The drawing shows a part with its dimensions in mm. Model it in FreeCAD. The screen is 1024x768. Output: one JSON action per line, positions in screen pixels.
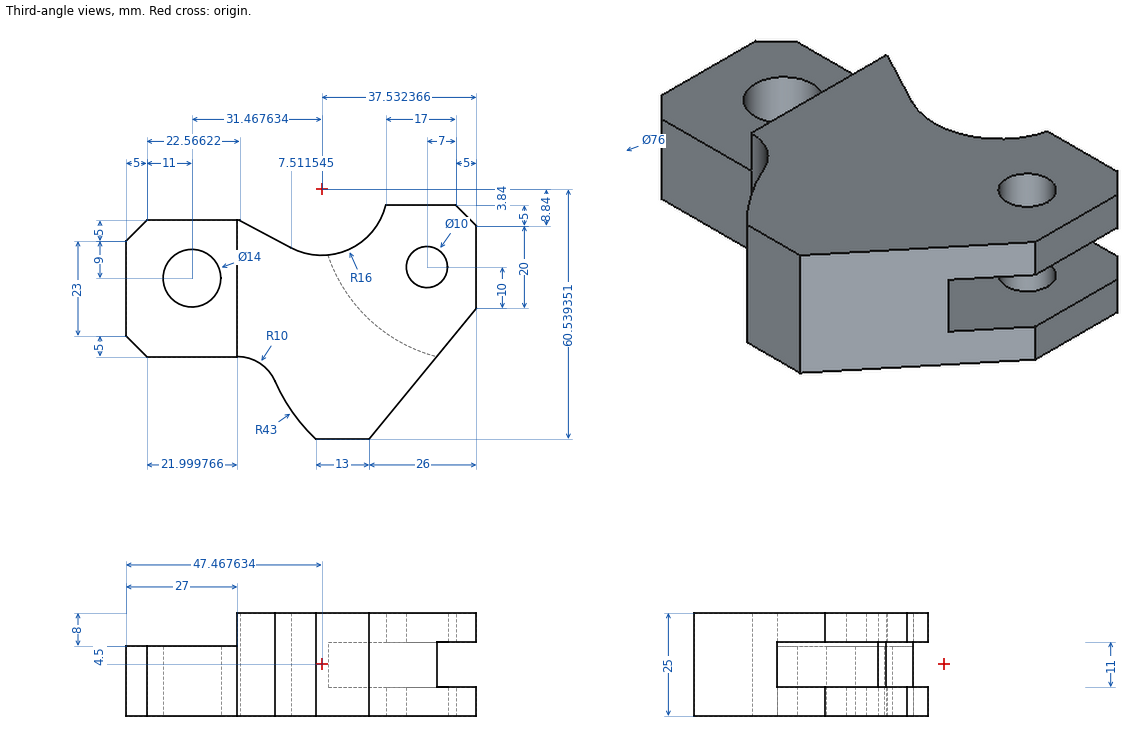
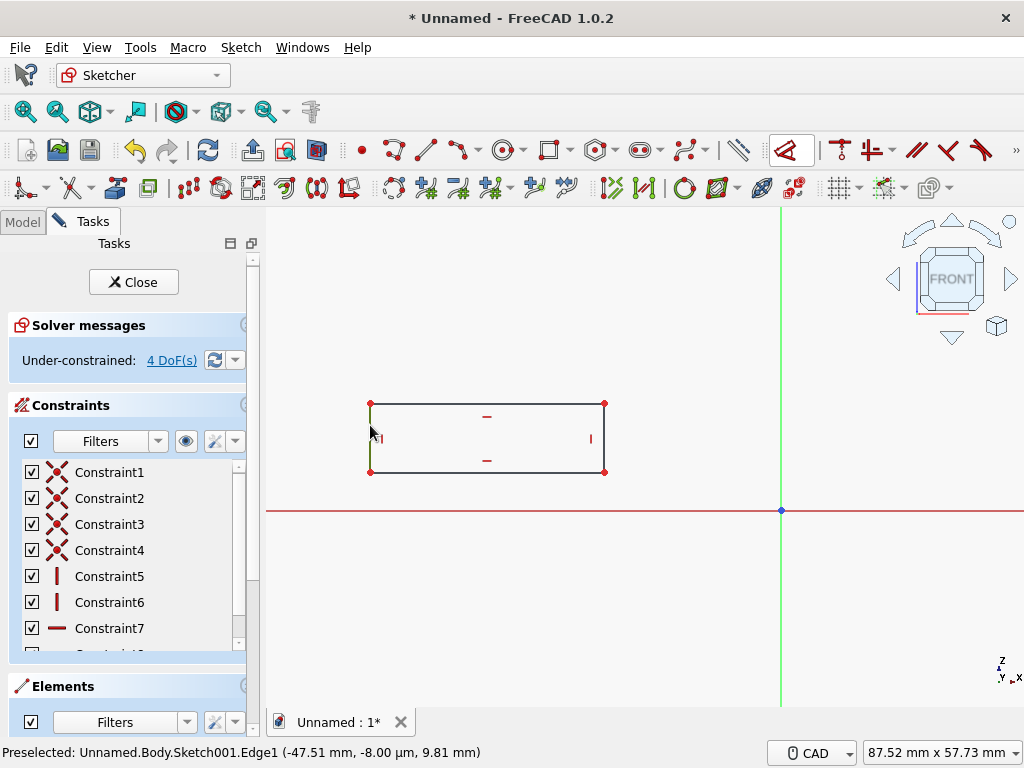
{"action": "left_click", "coordinate": [808, 150]}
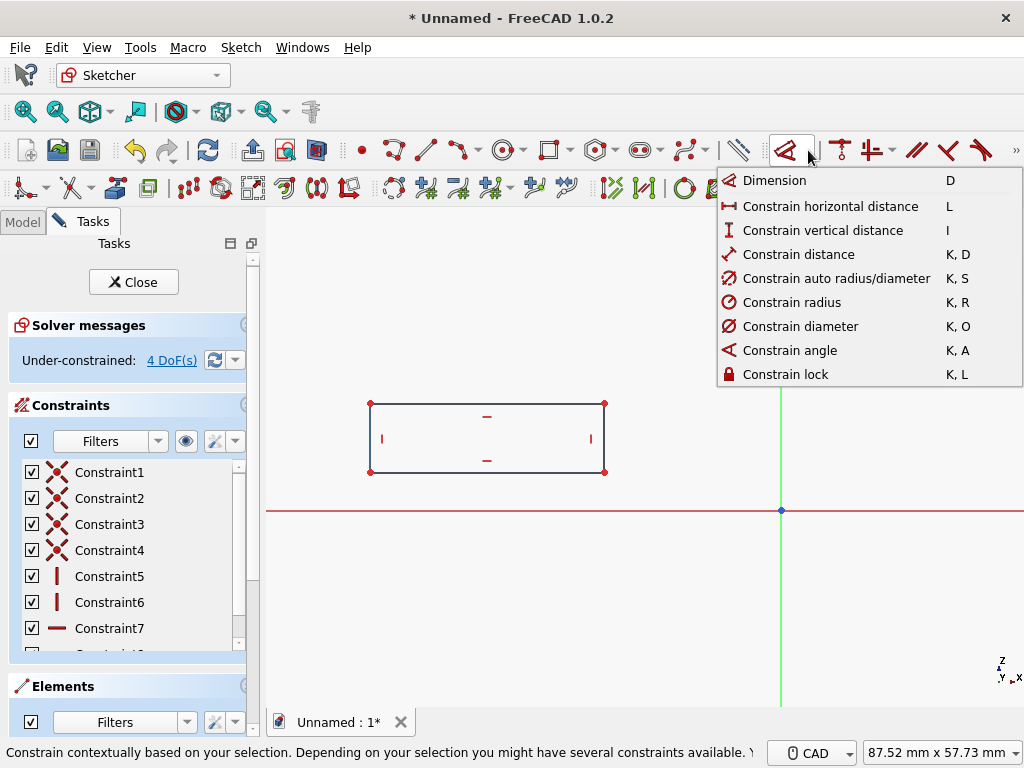
{"action": "left_click", "coordinate": [870, 230]}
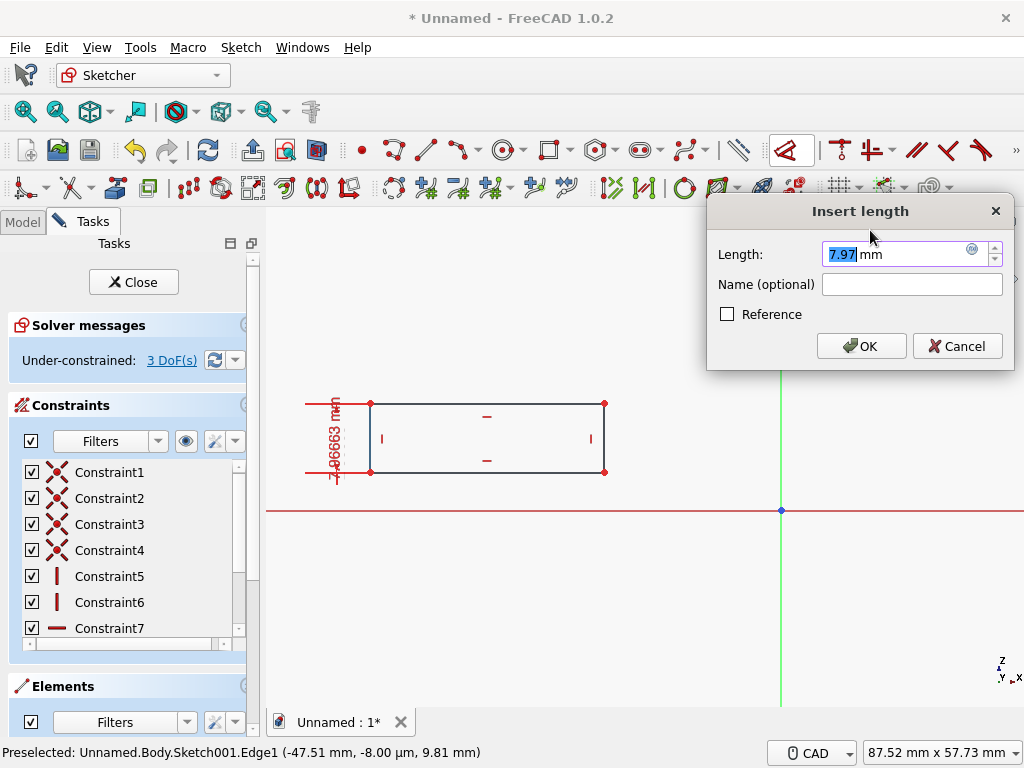
{"action": "type", "text": "8"}
{"action": "key", "text": "Return"}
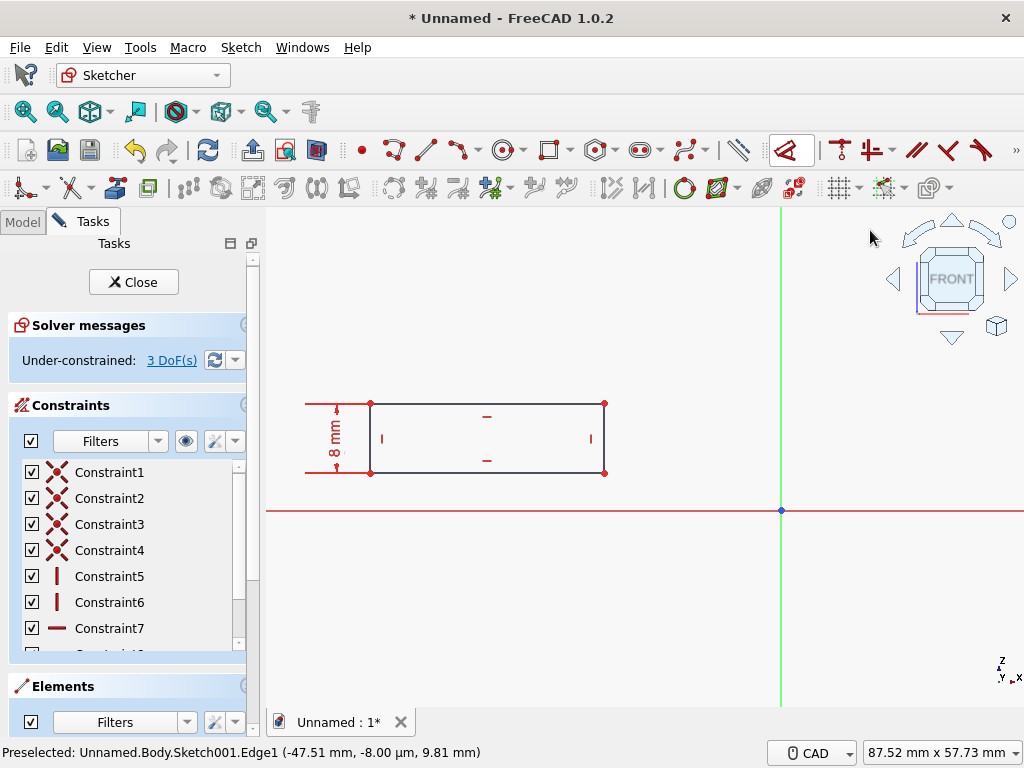
{"action": "left_click", "coordinate": [440, 473]}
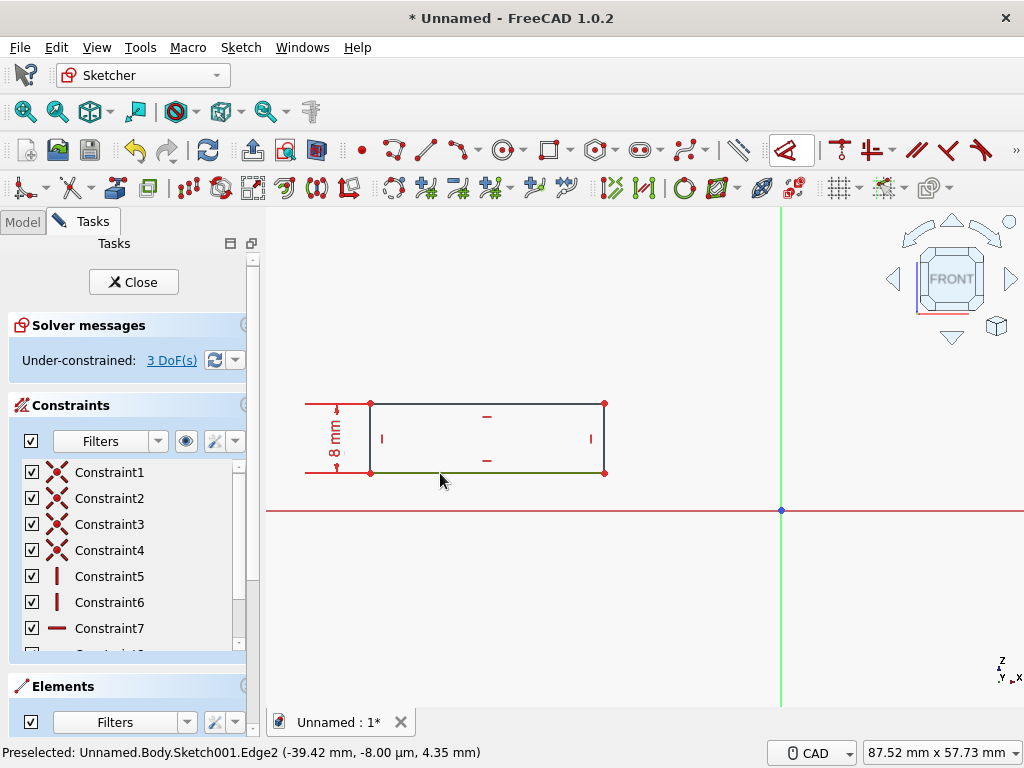
{"action": "key", "text": "l"}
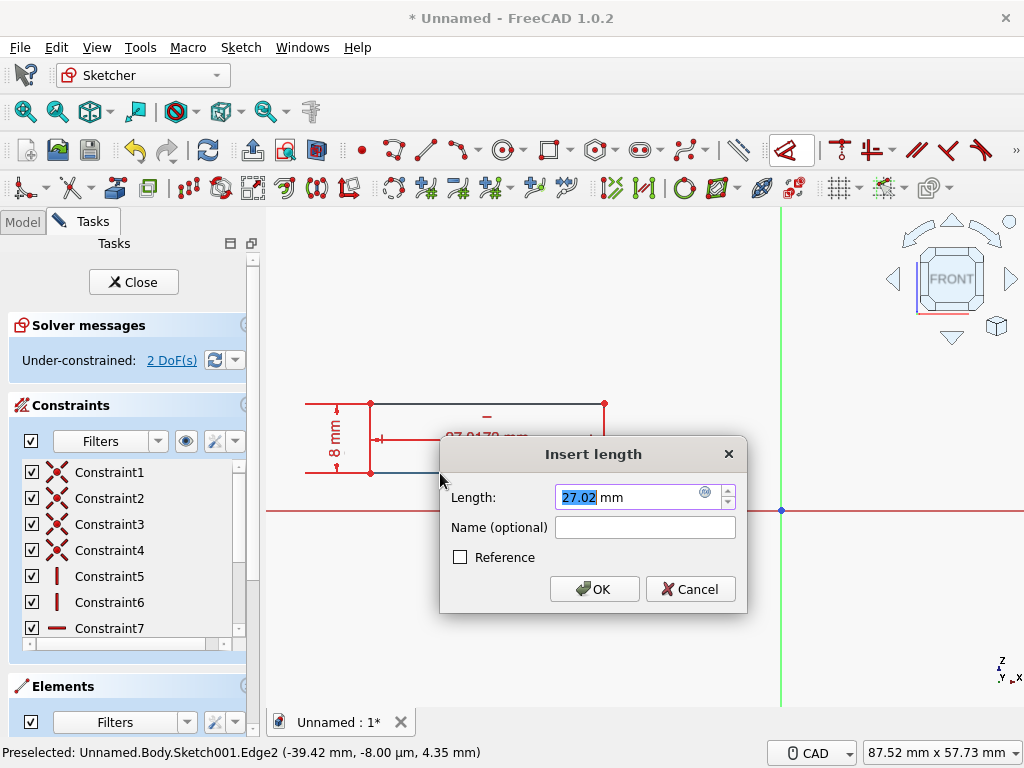
{"action": "type", "text": "27"}
{"action": "key", "text": "Return"}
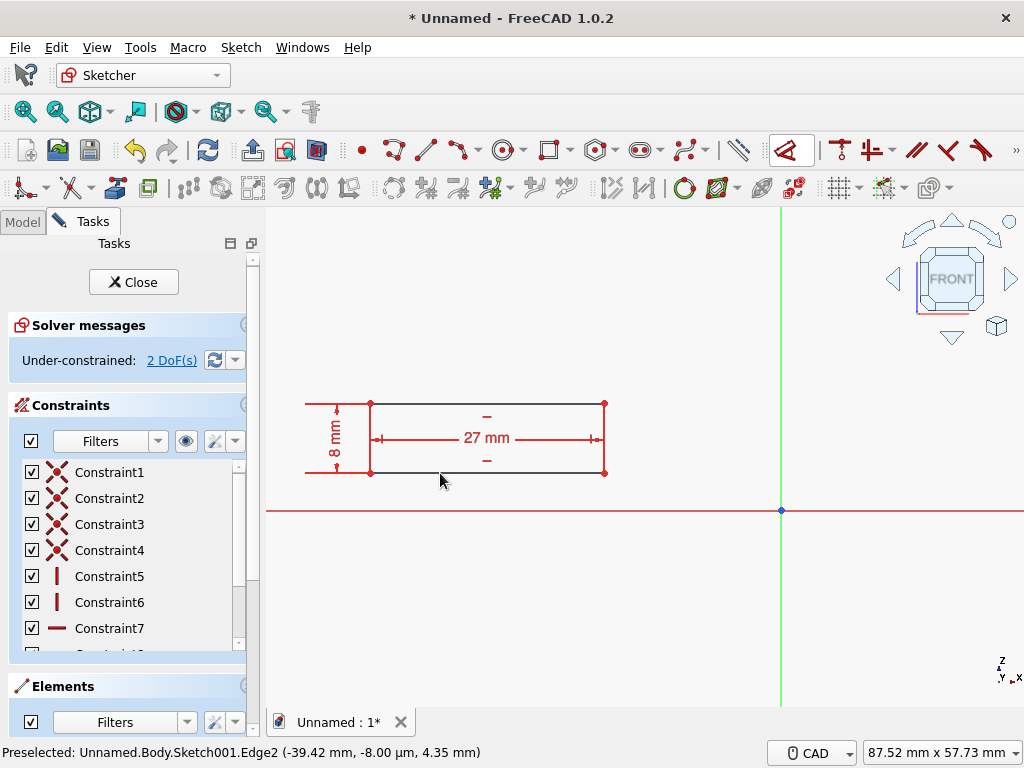
{"action": "left_click", "coordinate": [370, 473]}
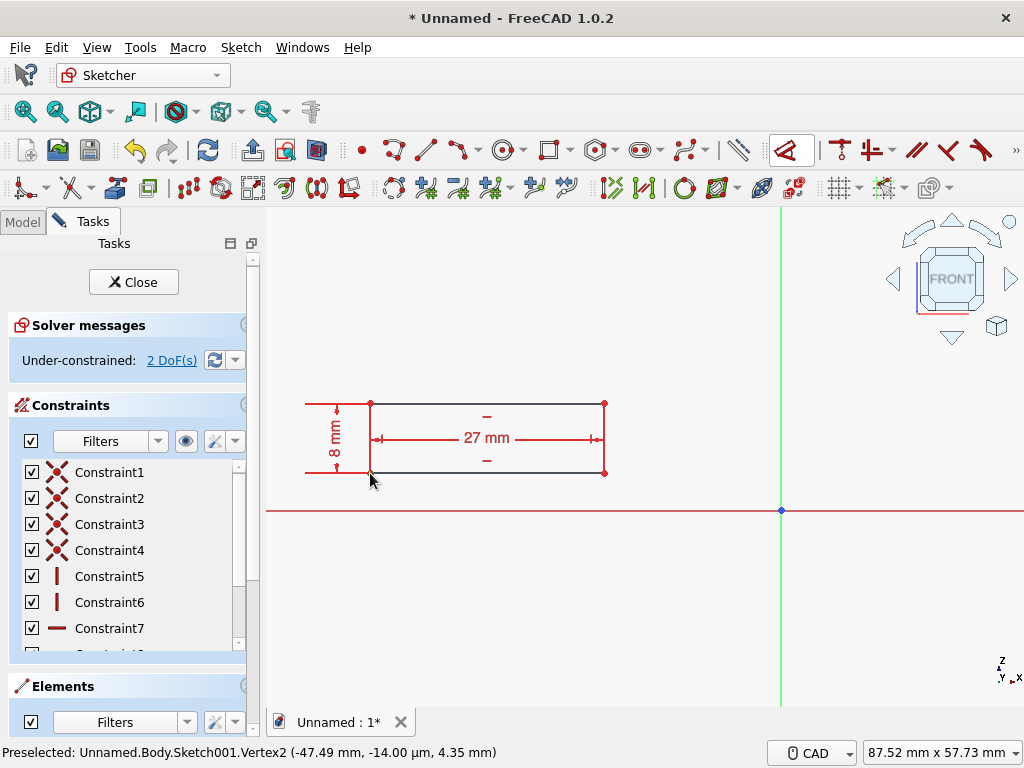
{"action": "key", "text": "i"}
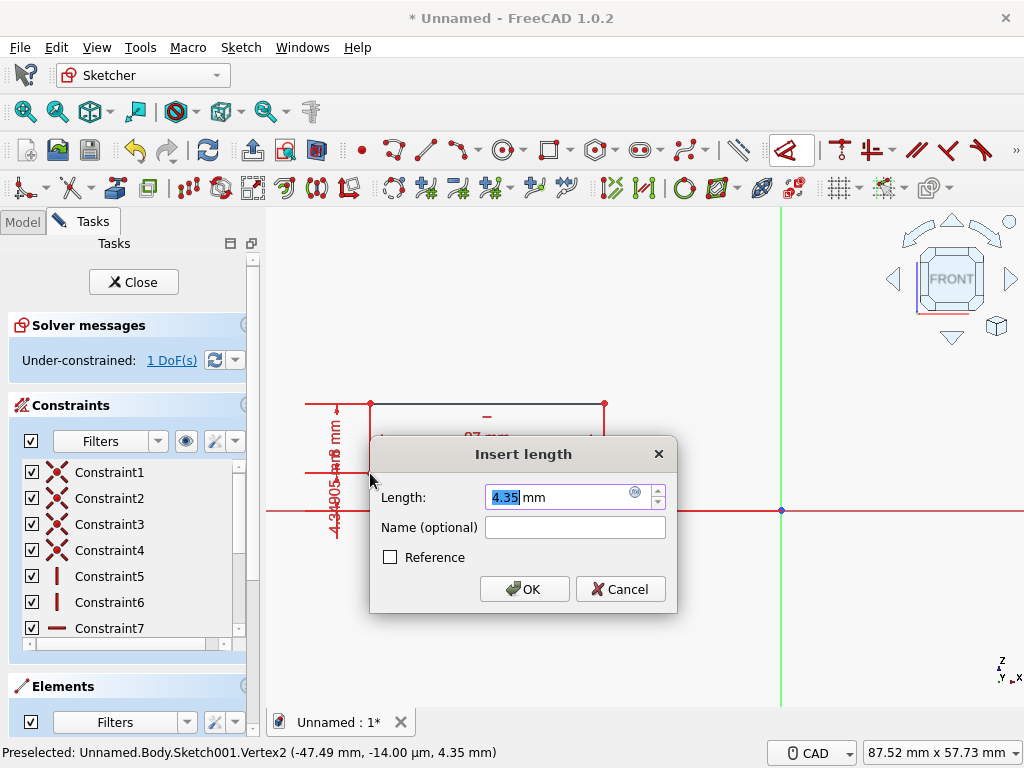
{"action": "type", "text": "4.5"}
{"action": "key", "text": "Return"}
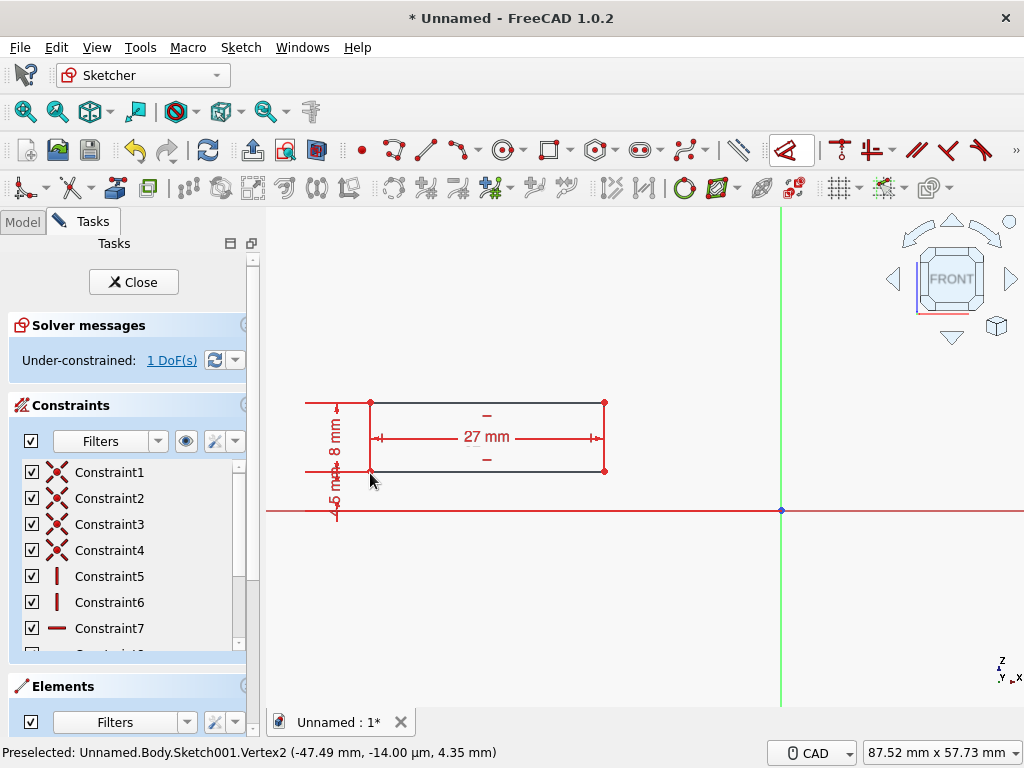
{"action": "left_click", "coordinate": [370, 403]}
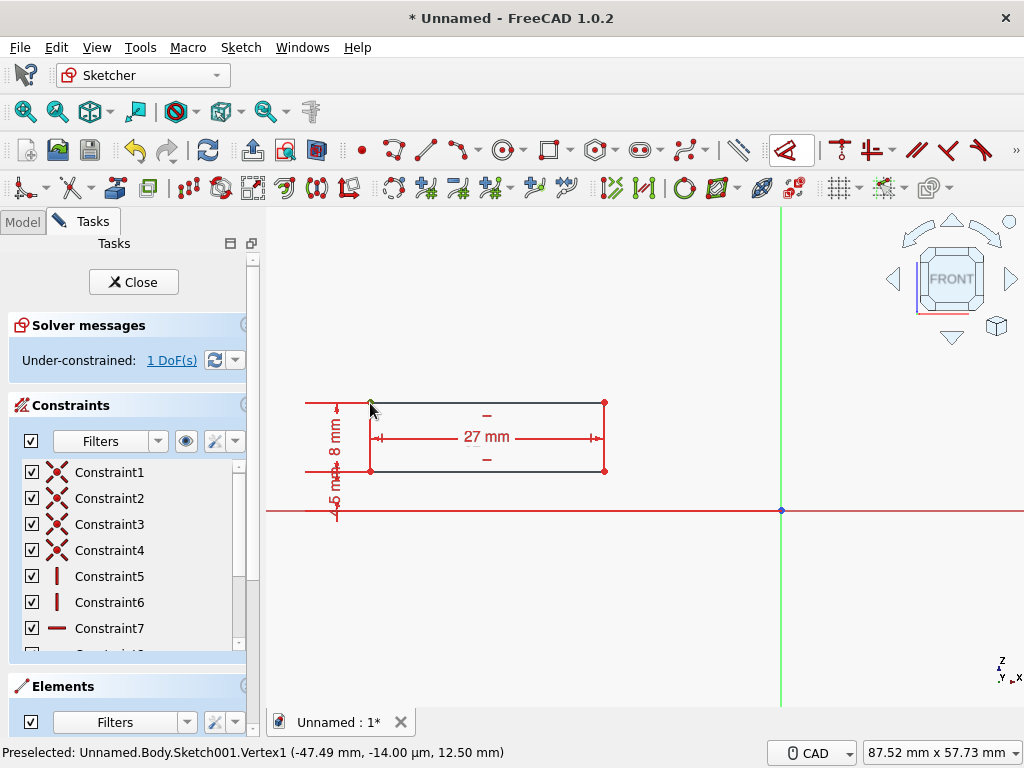
{"action": "key", "text": "l"}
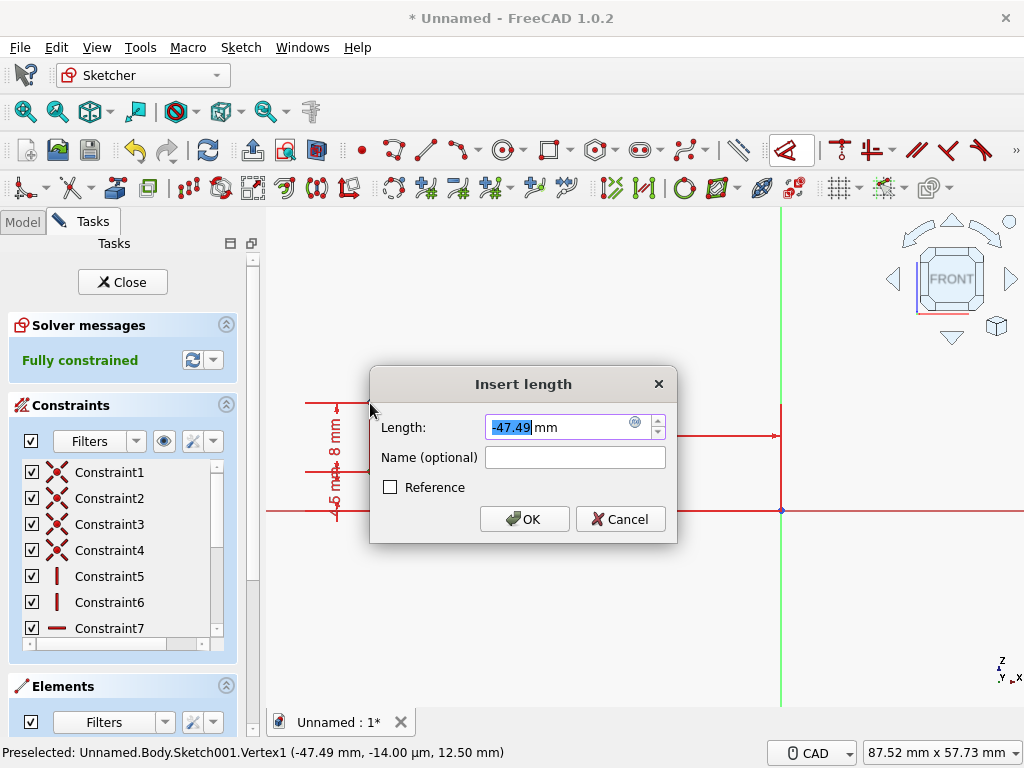
{"action": "type", "text": "-47.467634"}
{"action": "key", "text": "Return"}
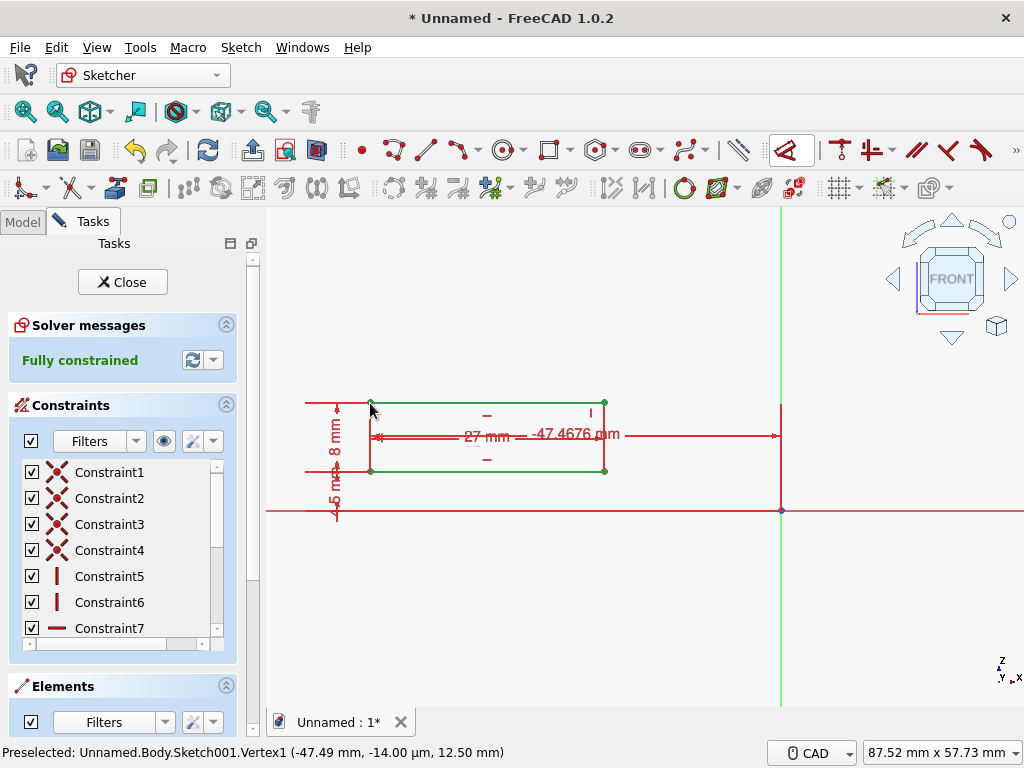
{"action": "left_click", "coordinate": [123, 282]}